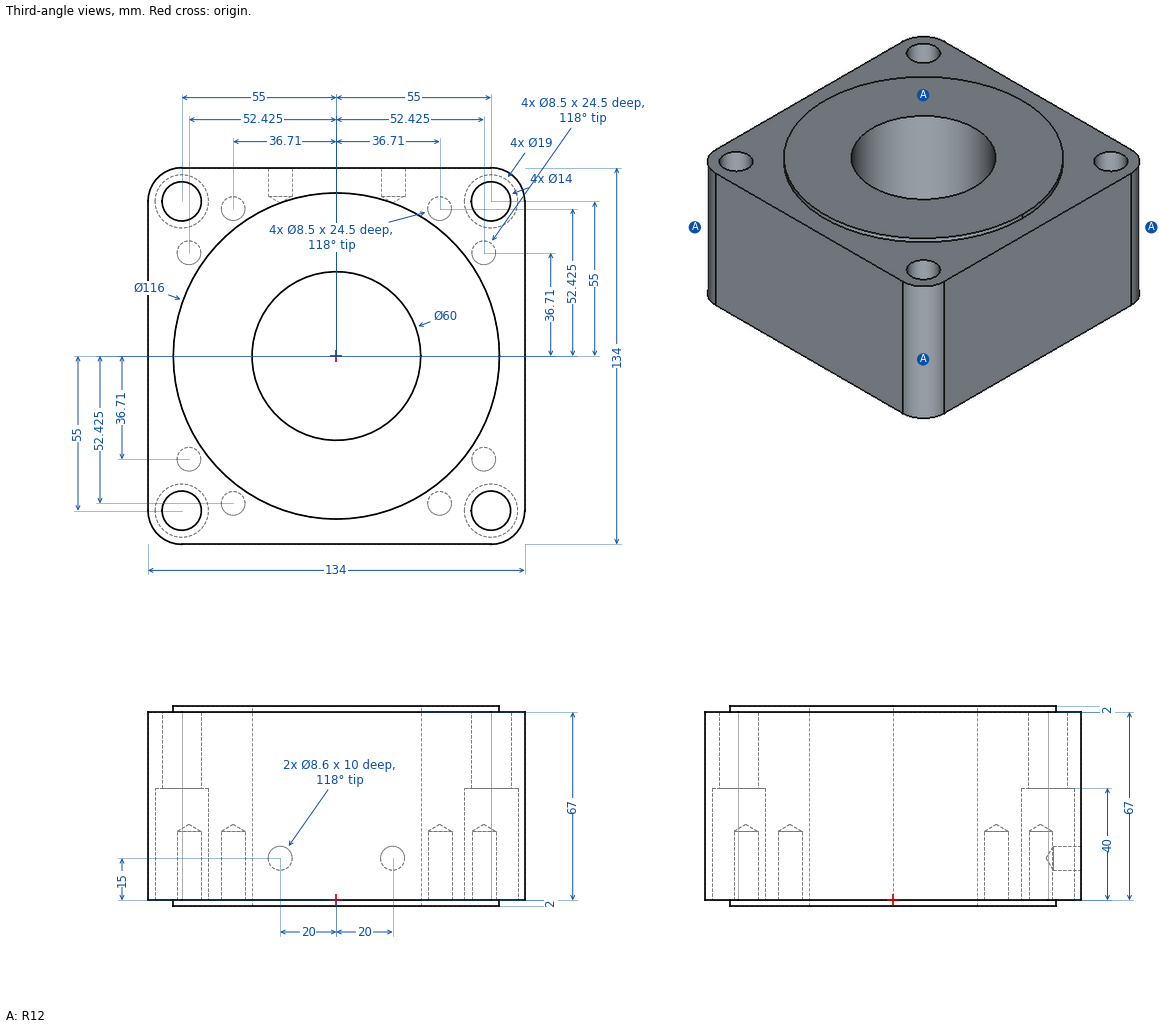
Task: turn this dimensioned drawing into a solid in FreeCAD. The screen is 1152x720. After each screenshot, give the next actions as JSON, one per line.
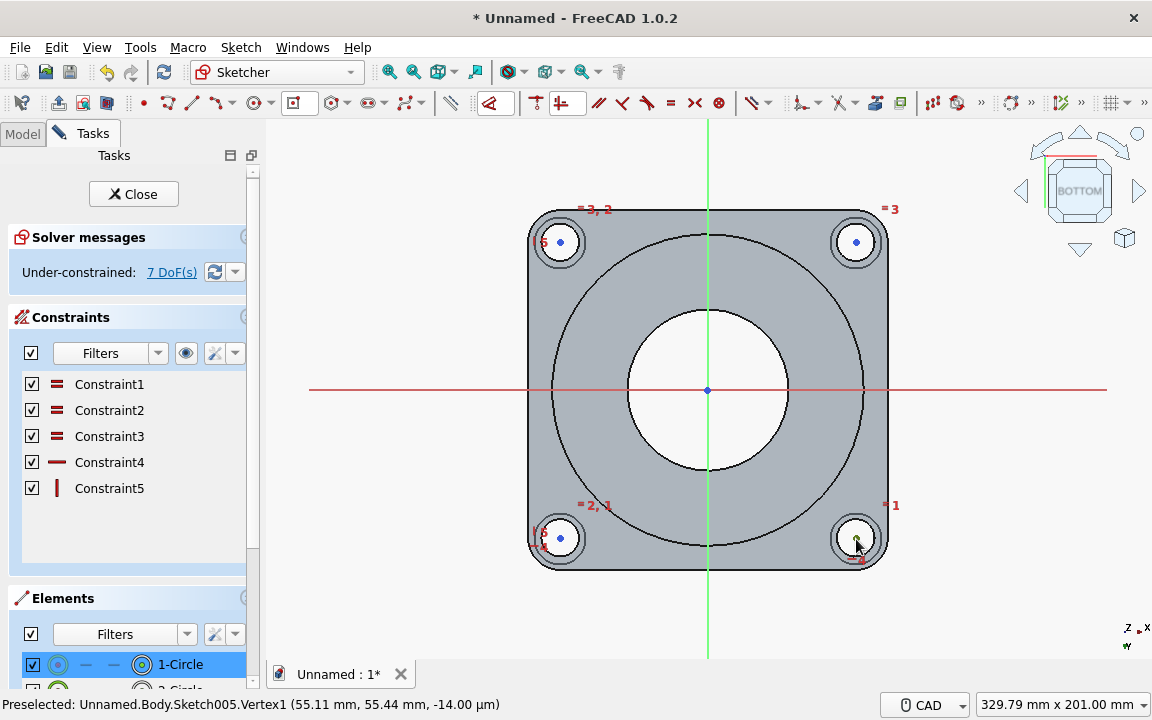
{"action": "left_click", "coordinate": [856, 243]}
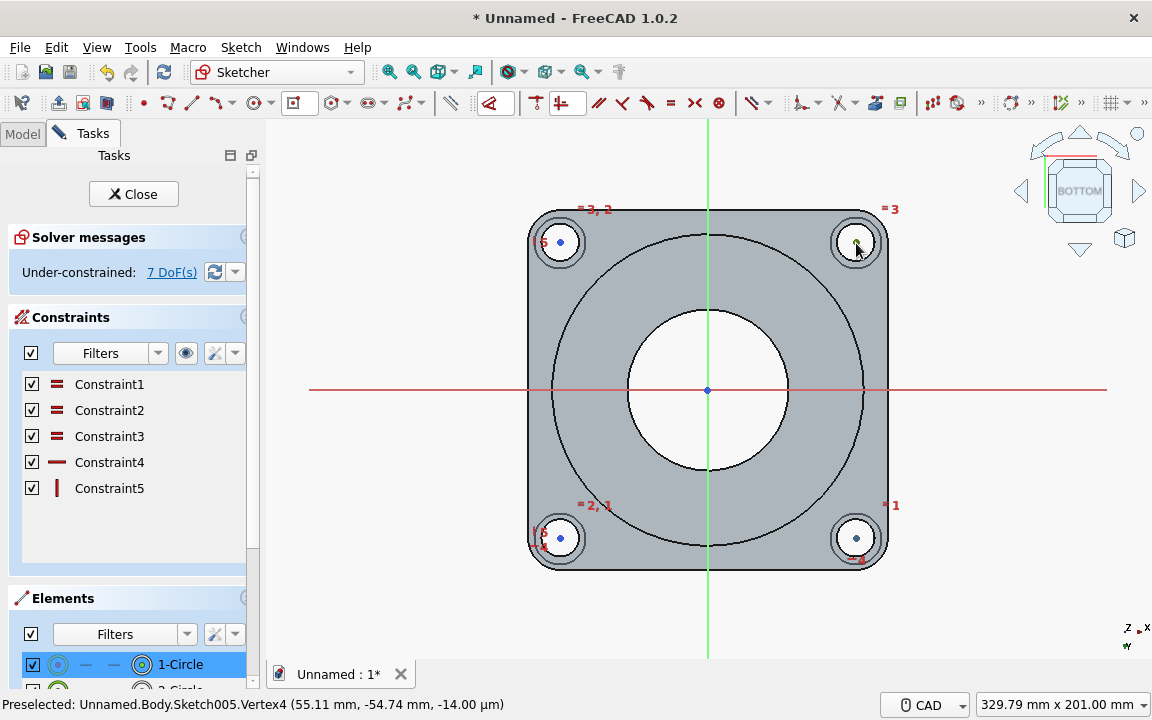
{"action": "key", "text": "v"}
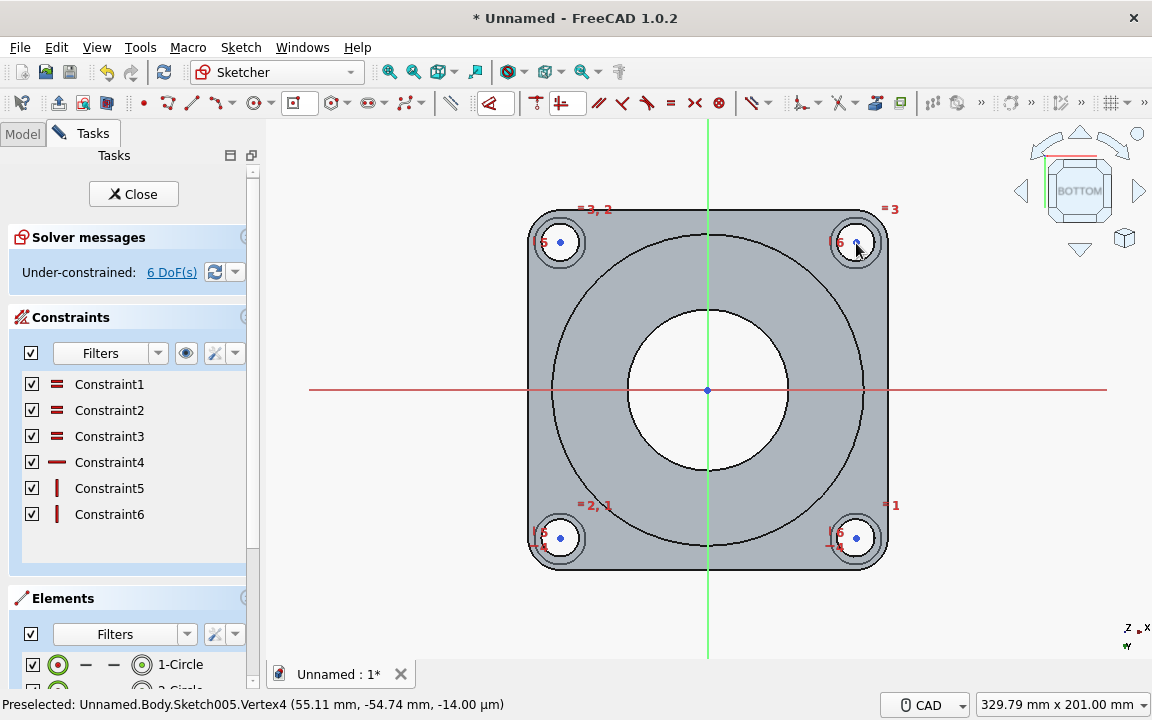
{"action": "left_click", "coordinate": [560, 243]}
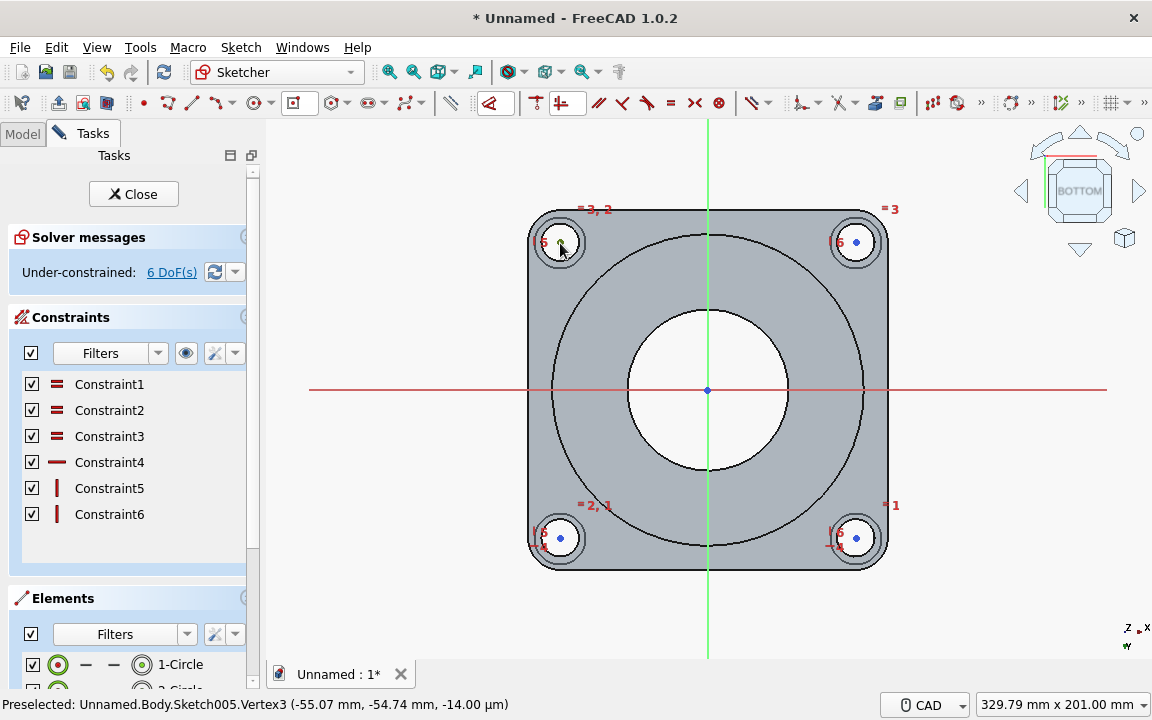
{"action": "left_click", "coordinate": [856, 243]}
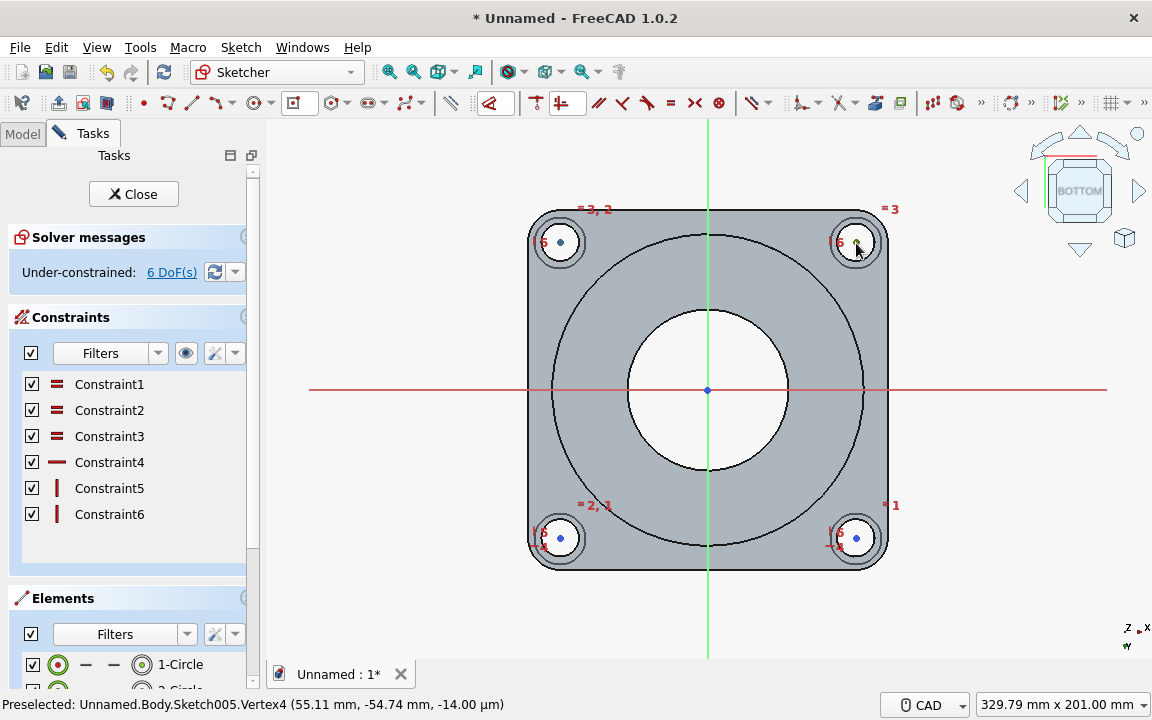
{"action": "key", "text": "h"}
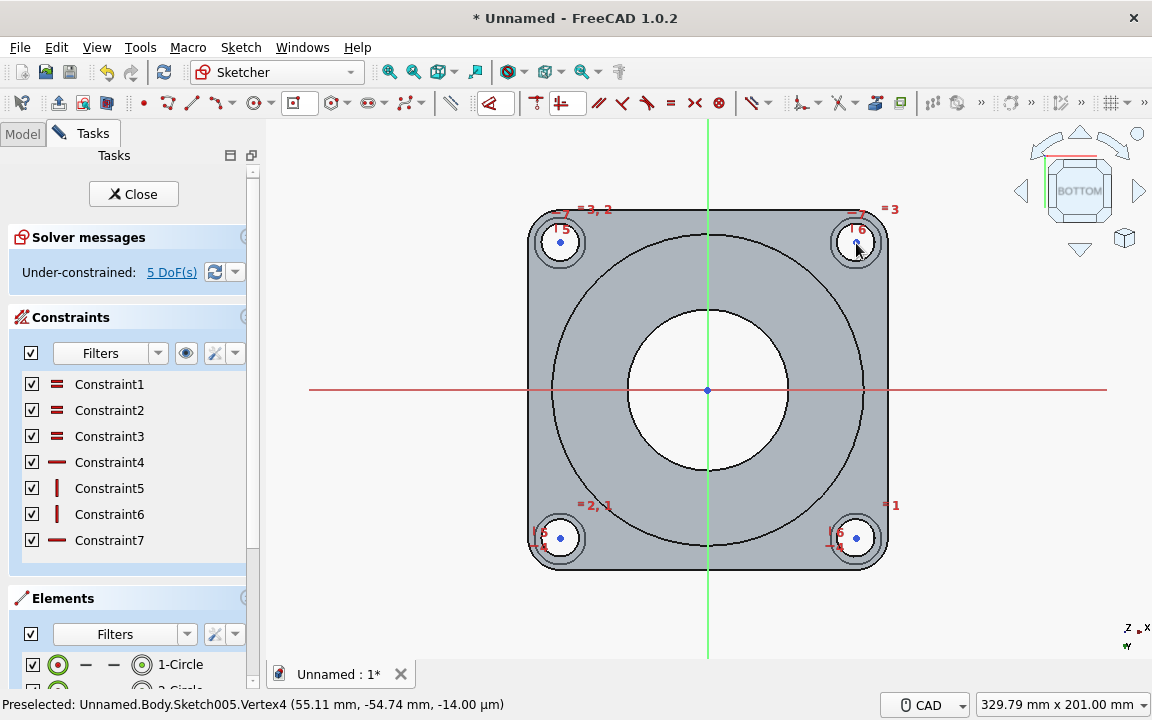
{"action": "left_click", "coordinate": [874, 521]}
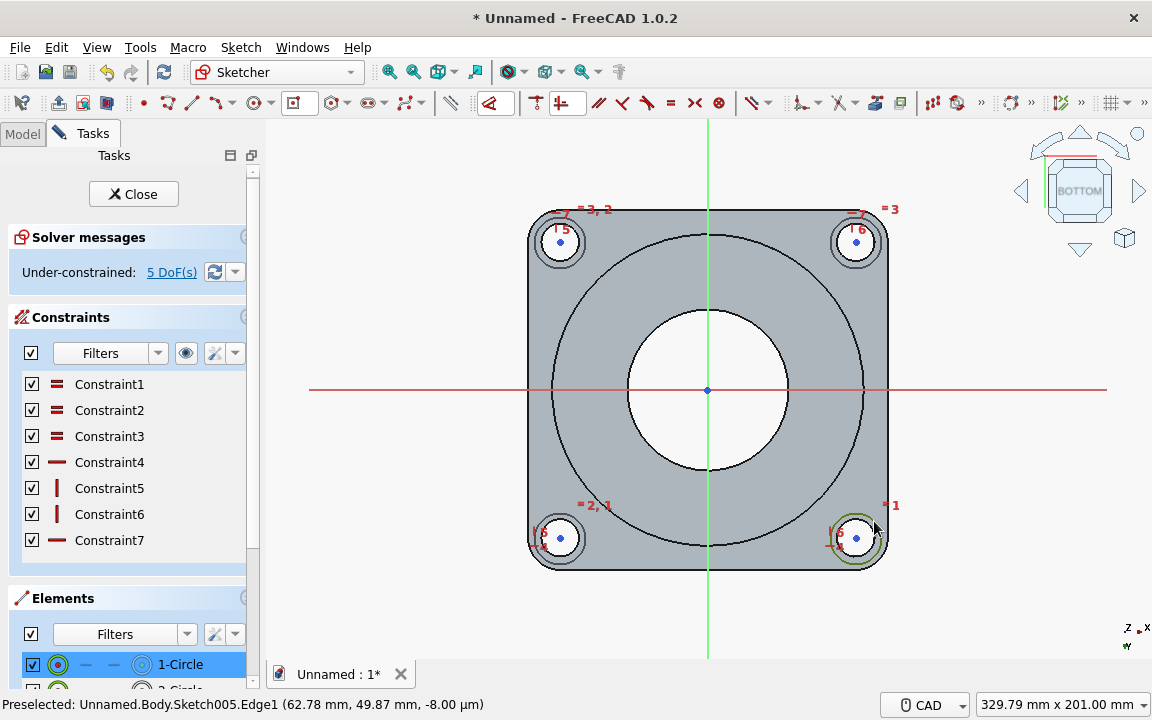
{"action": "key", "text": "k o"}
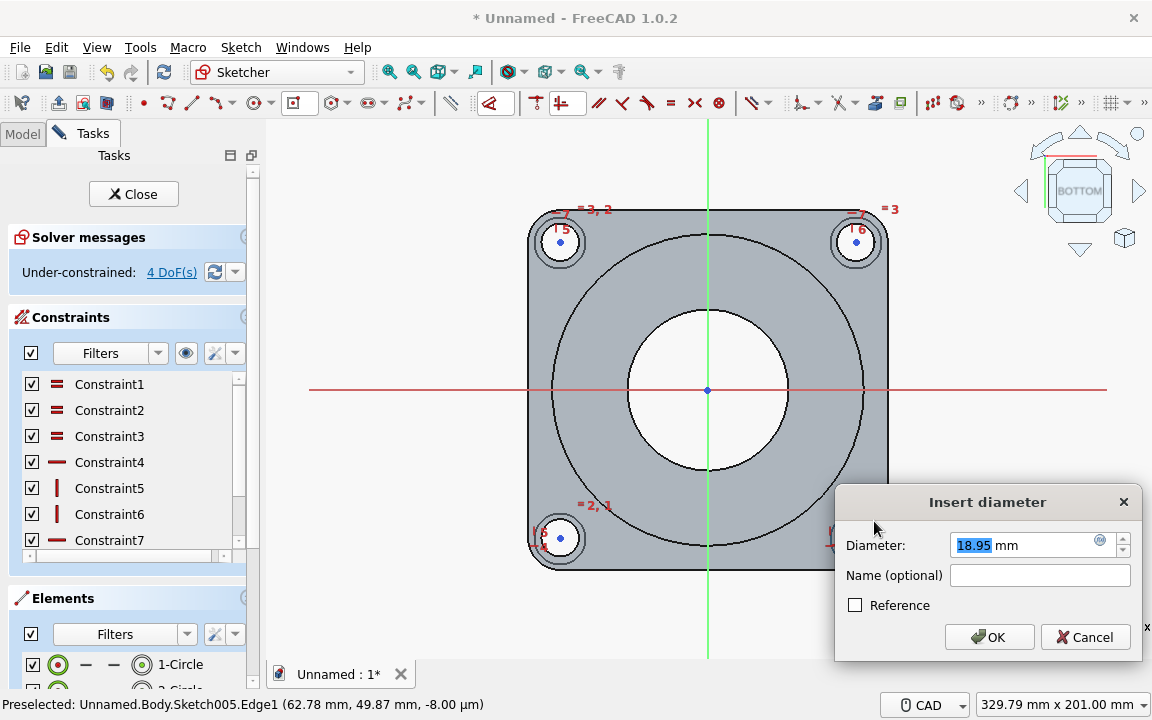
{"action": "type", "text": "19"}
{"action": "key", "text": "Return"}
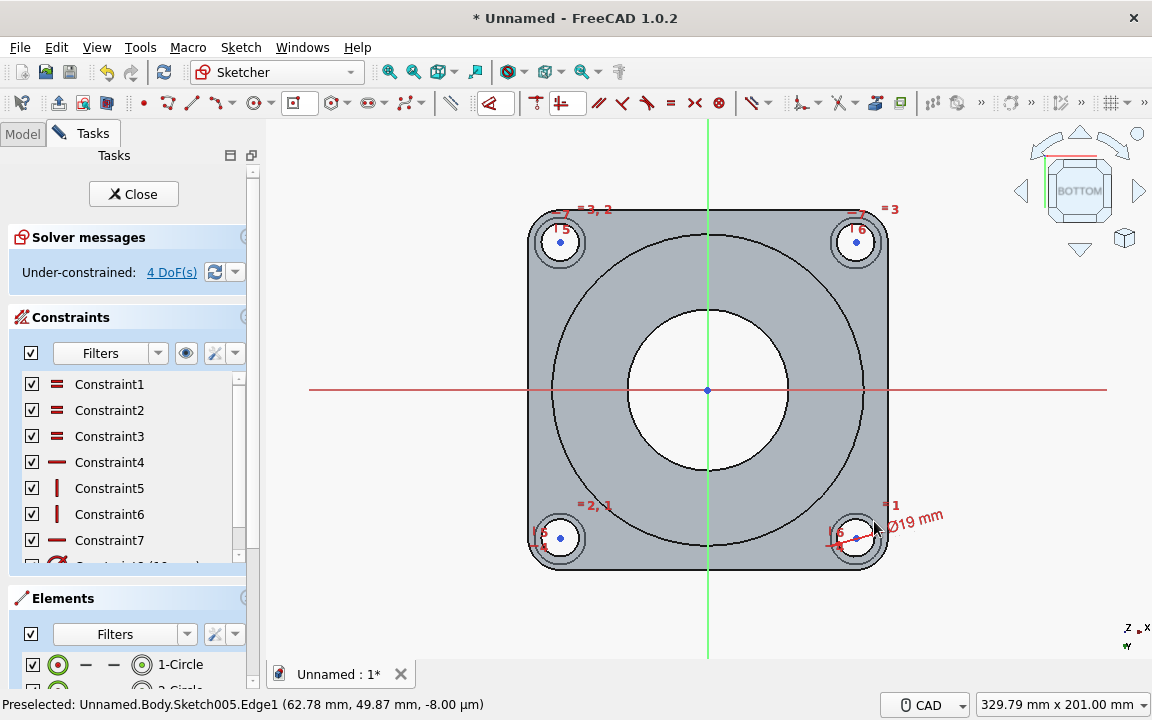
{"action": "left_click", "coordinate": [856, 539]}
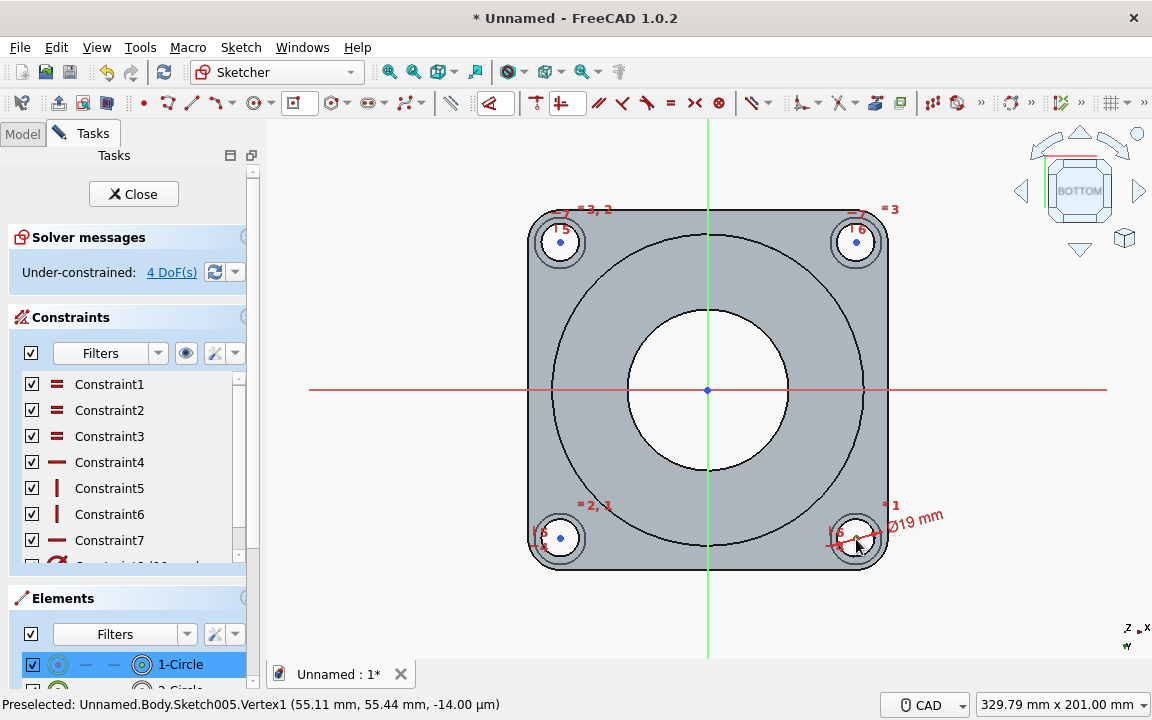
{"action": "left_click", "coordinate": [508, 104]}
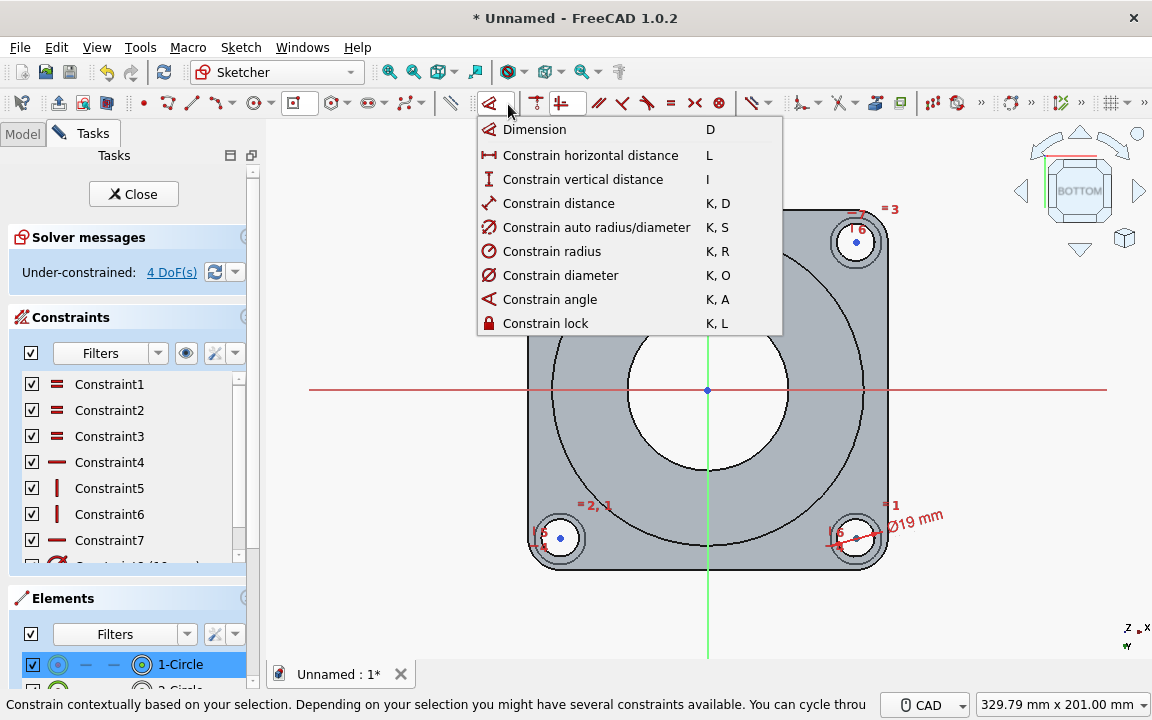
{"action": "left_click", "coordinate": [630, 155]}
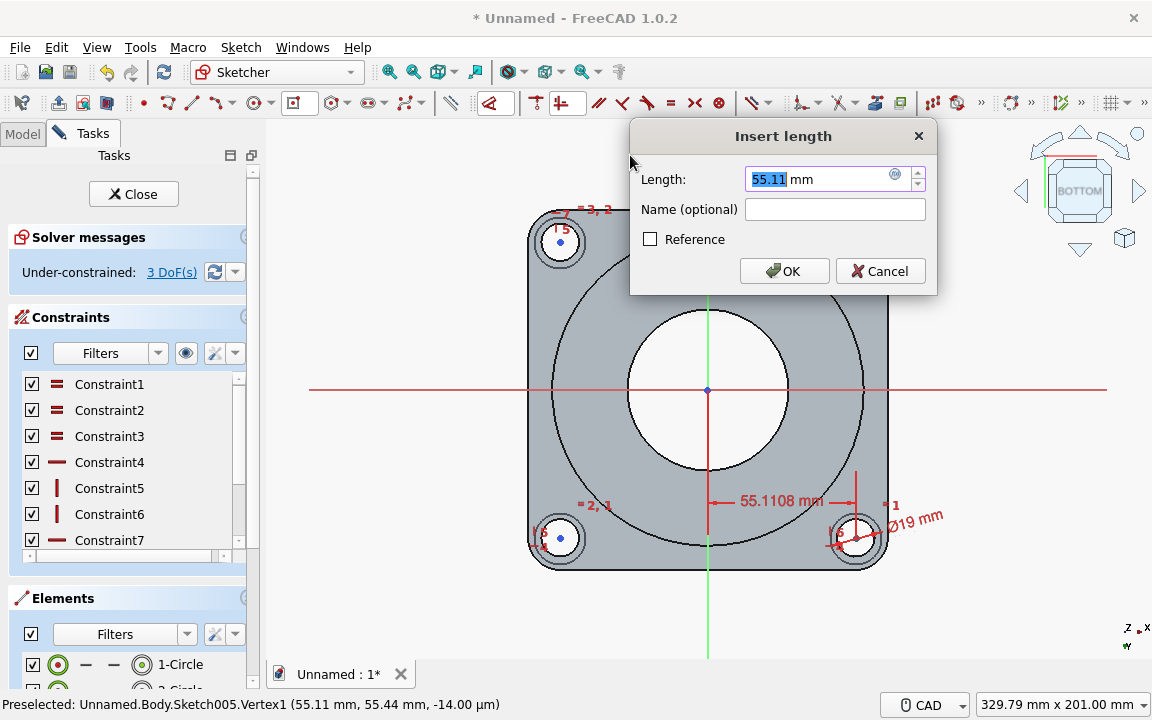
{"action": "type", "text": "55"}
{"action": "key", "text": "Return"}